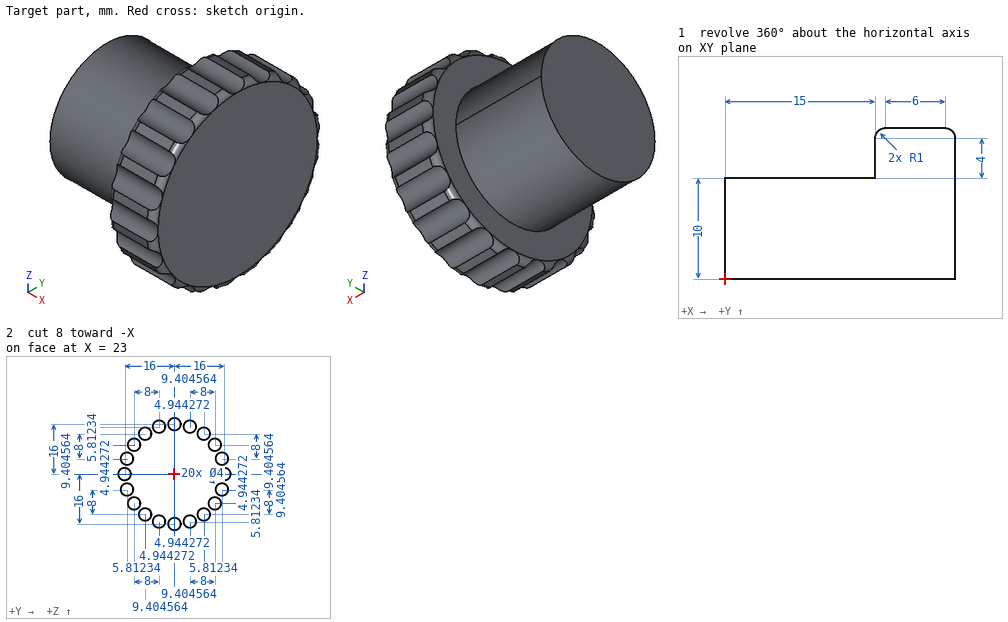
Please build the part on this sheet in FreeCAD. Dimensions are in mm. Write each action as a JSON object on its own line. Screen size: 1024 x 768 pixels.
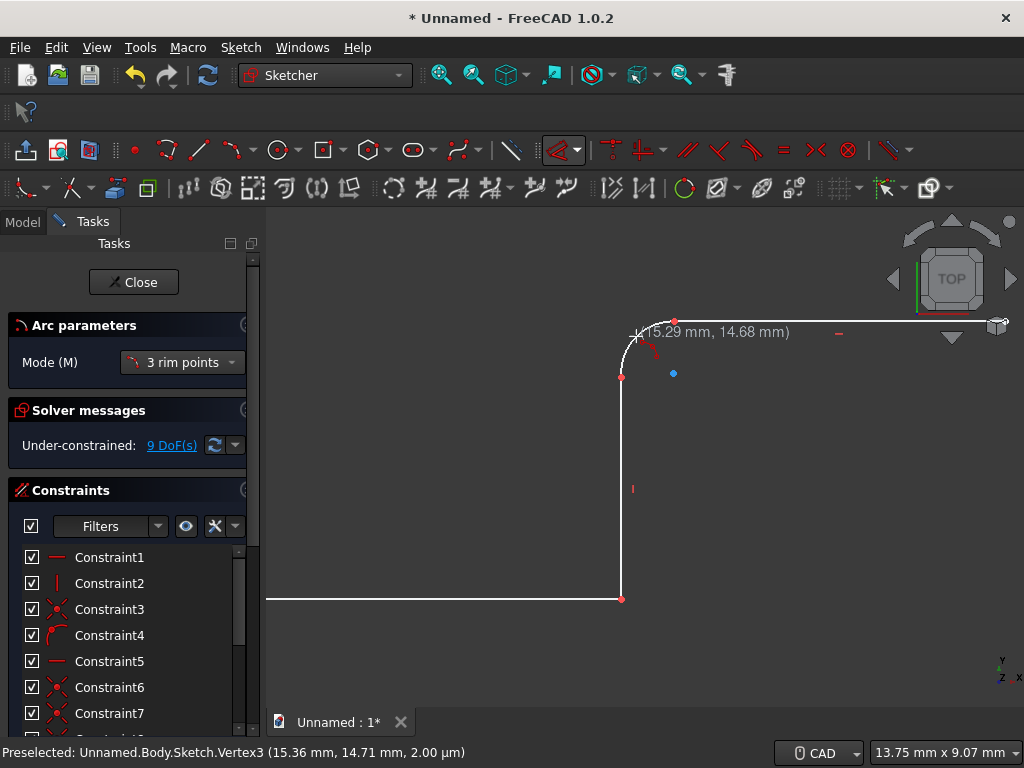
{"action": "scroll", "coordinate": [641, 338], "scroll_direction": "down", "scroll_amount": 6}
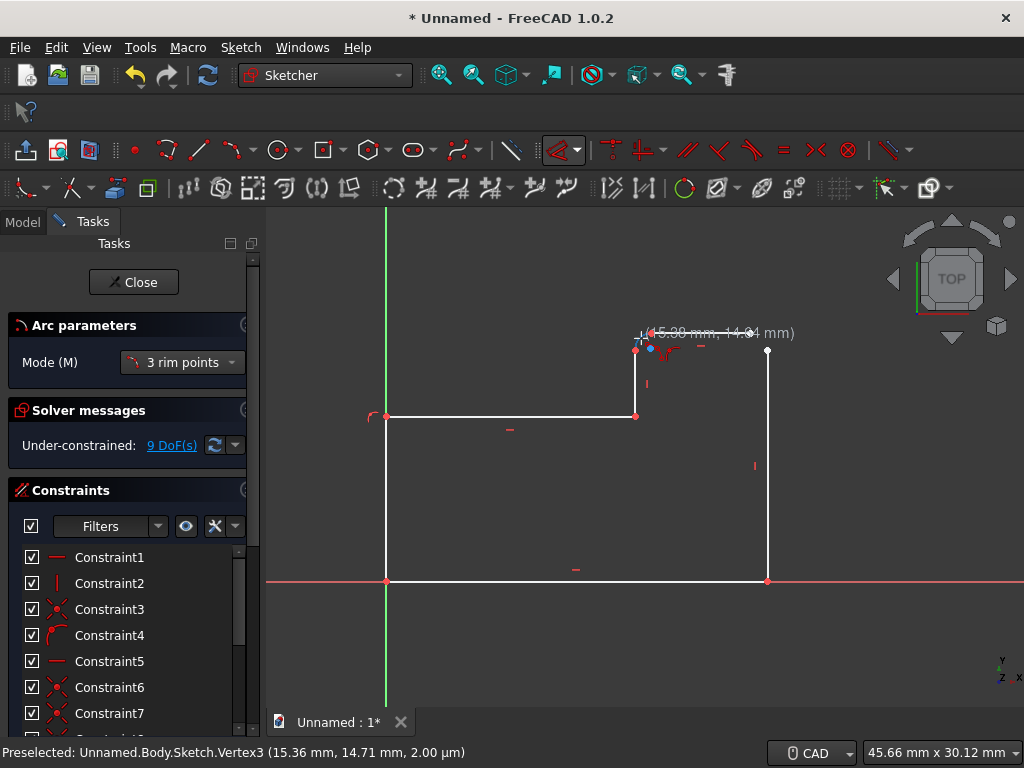
{"action": "left_click", "coordinate": [768, 350]}
{"action": "left_click", "coordinate": [751, 333]}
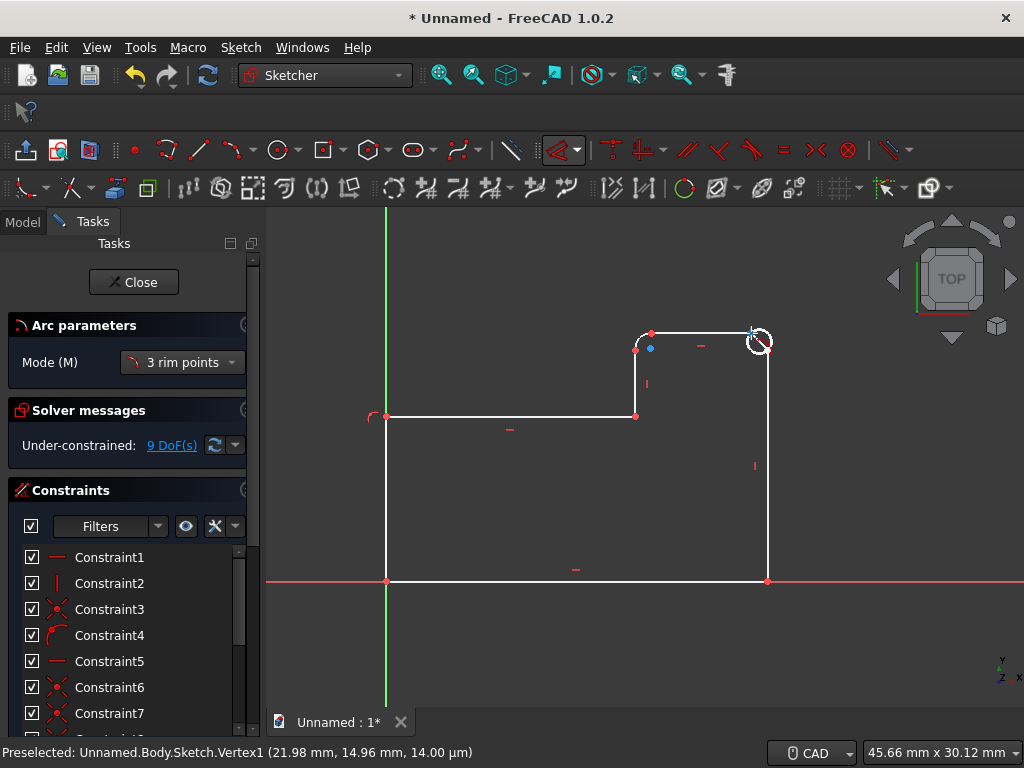
{"action": "scroll", "coordinate": [763, 337], "scroll_direction": "up", "scroll_amount": 6}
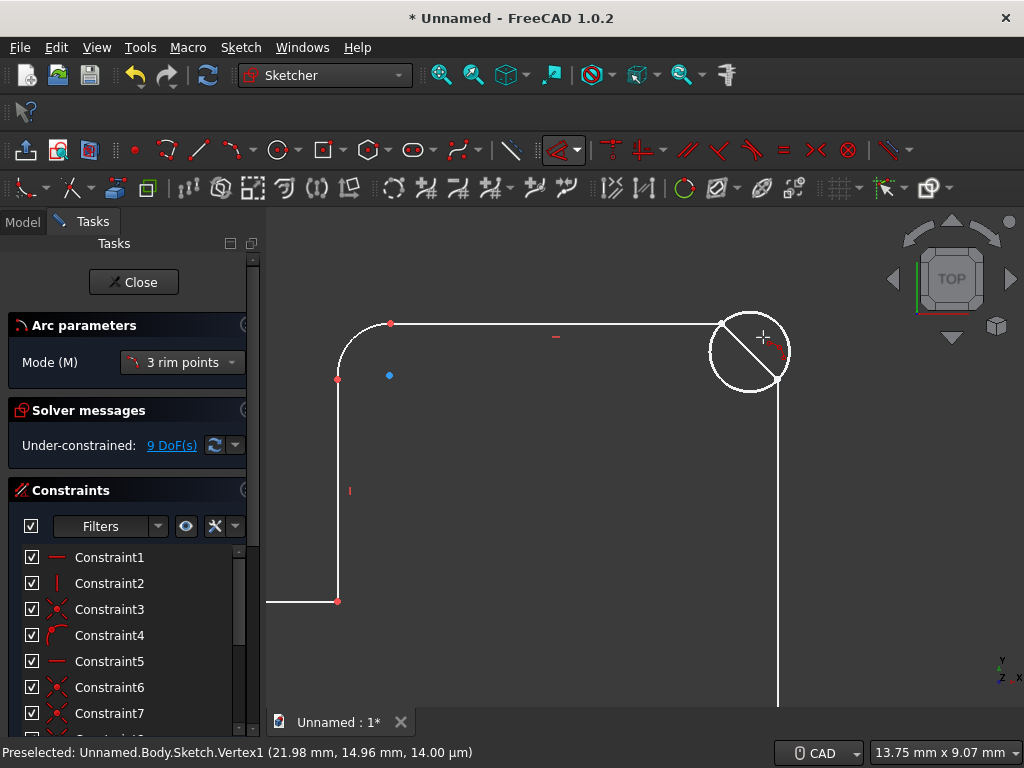
{"action": "left_click", "coordinate": [762, 338]}
{"action": "key", "text": "Escape"}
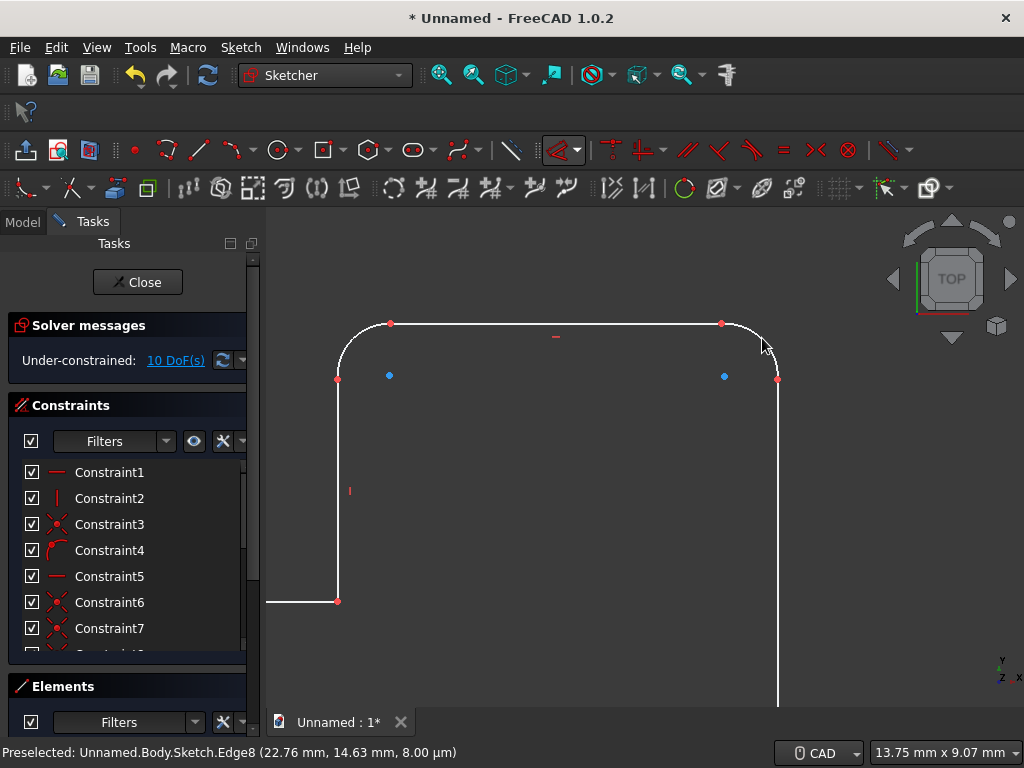
{"action": "left_click", "coordinate": [622, 324]}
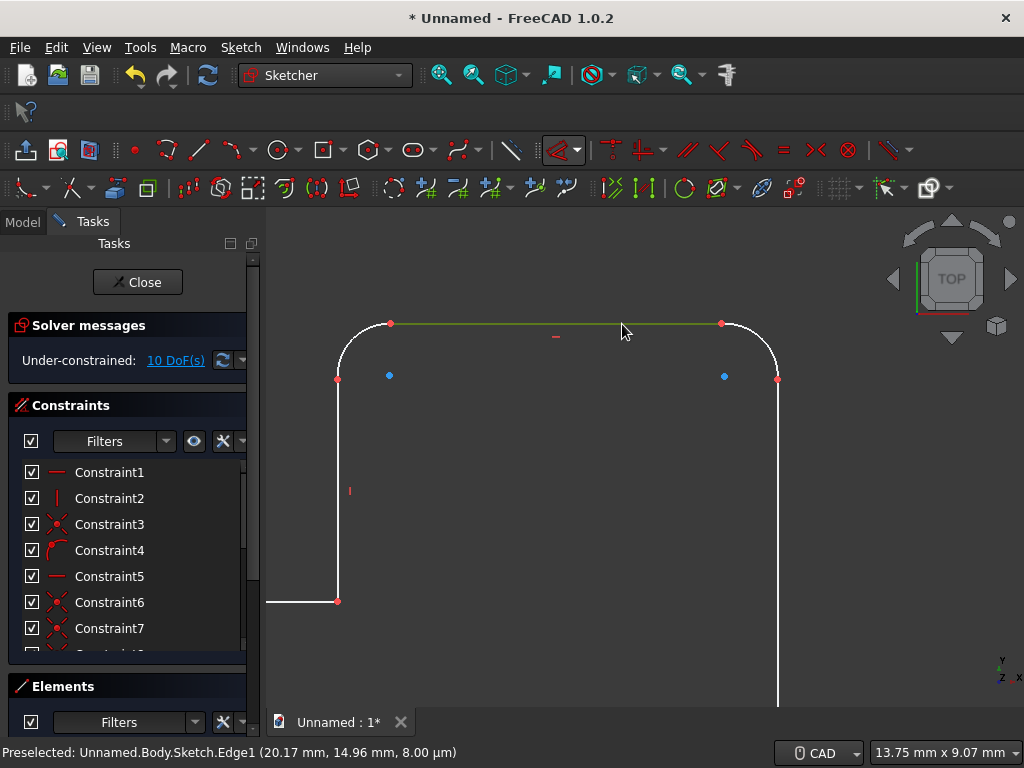
{"action": "left_click", "coordinate": [366, 330]}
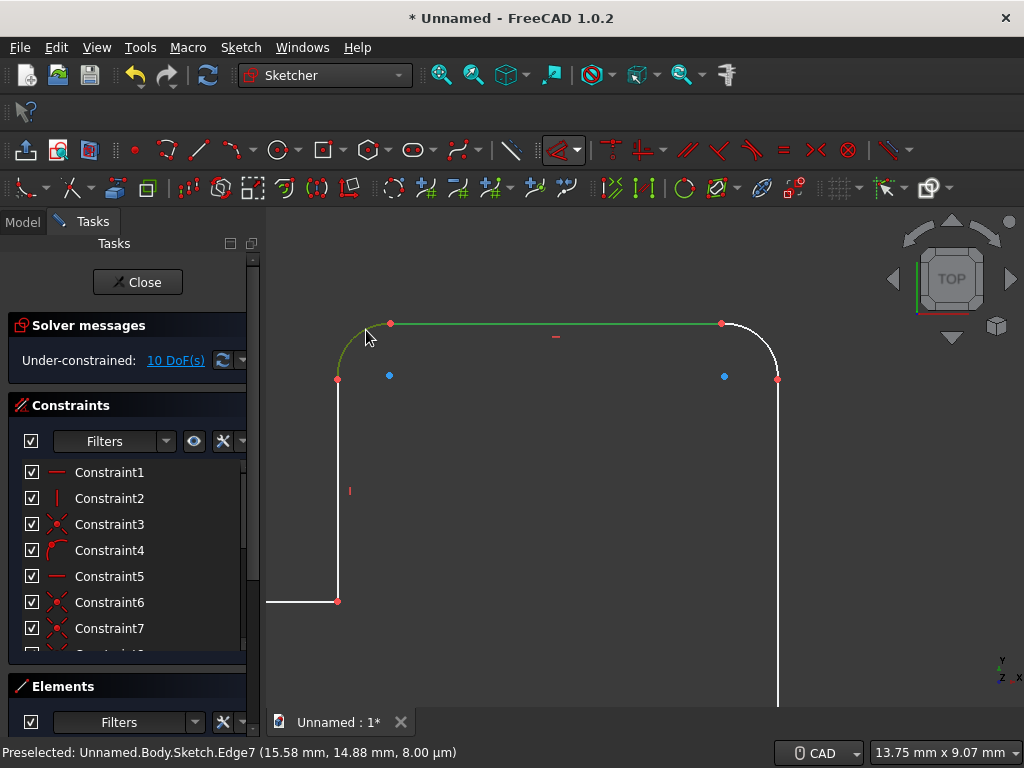
{"action": "left_click", "coordinate": [752, 150]}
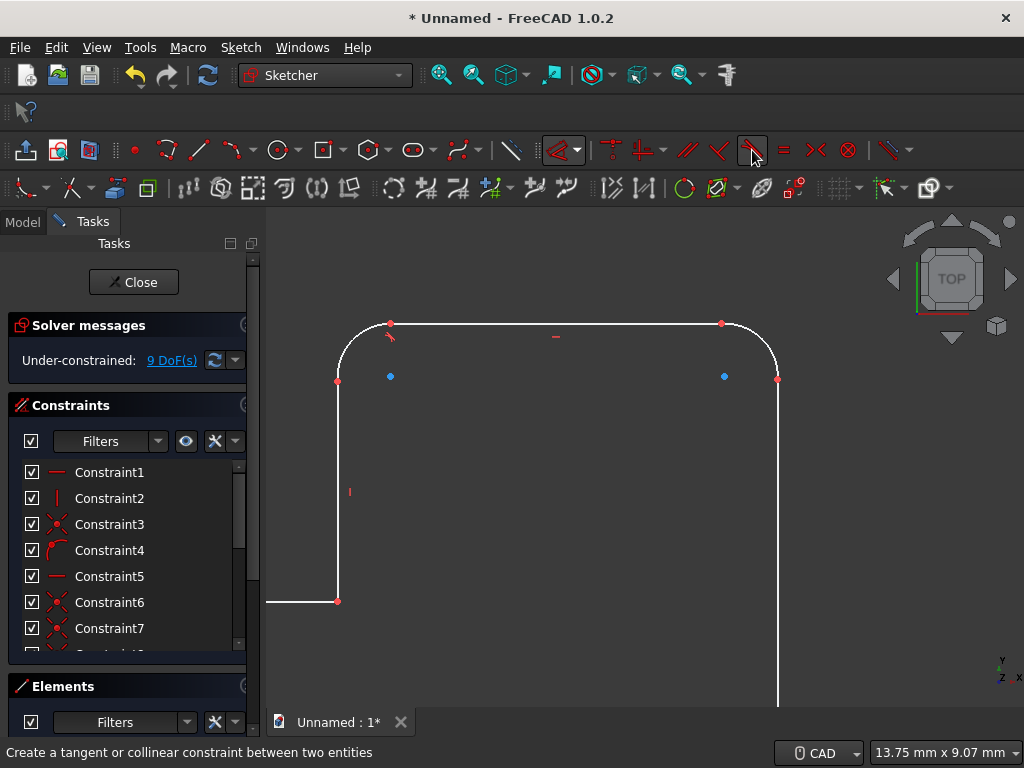
{"action": "left_click", "coordinate": [622, 324]}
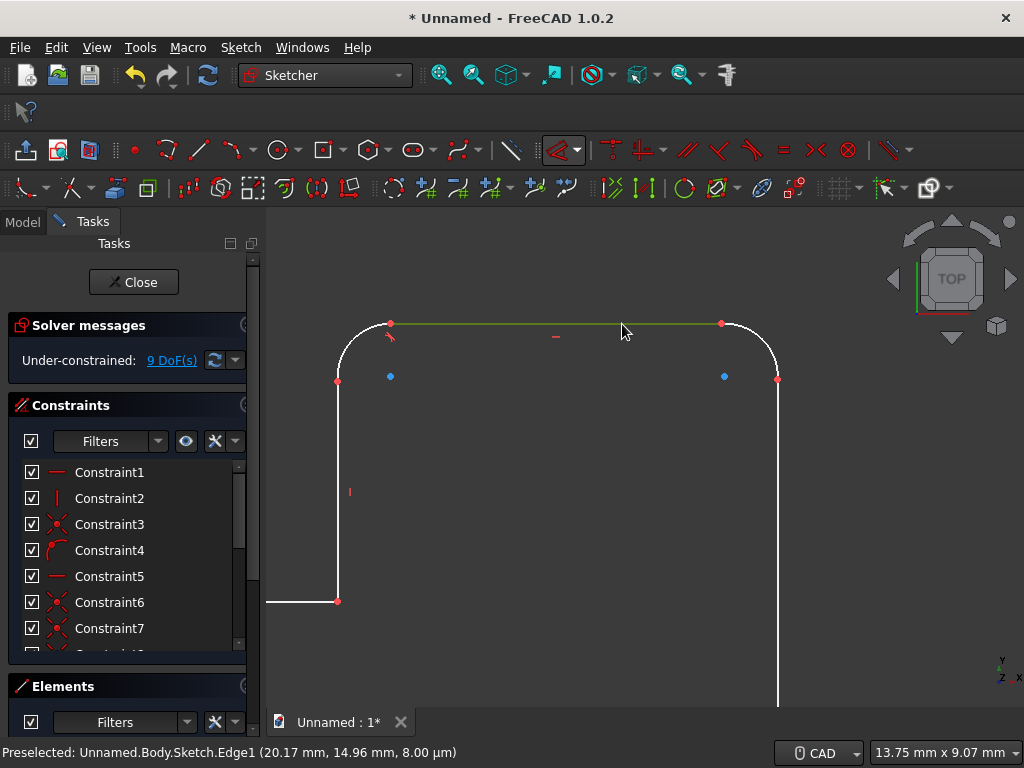
{"action": "left_click", "coordinate": [773, 354]}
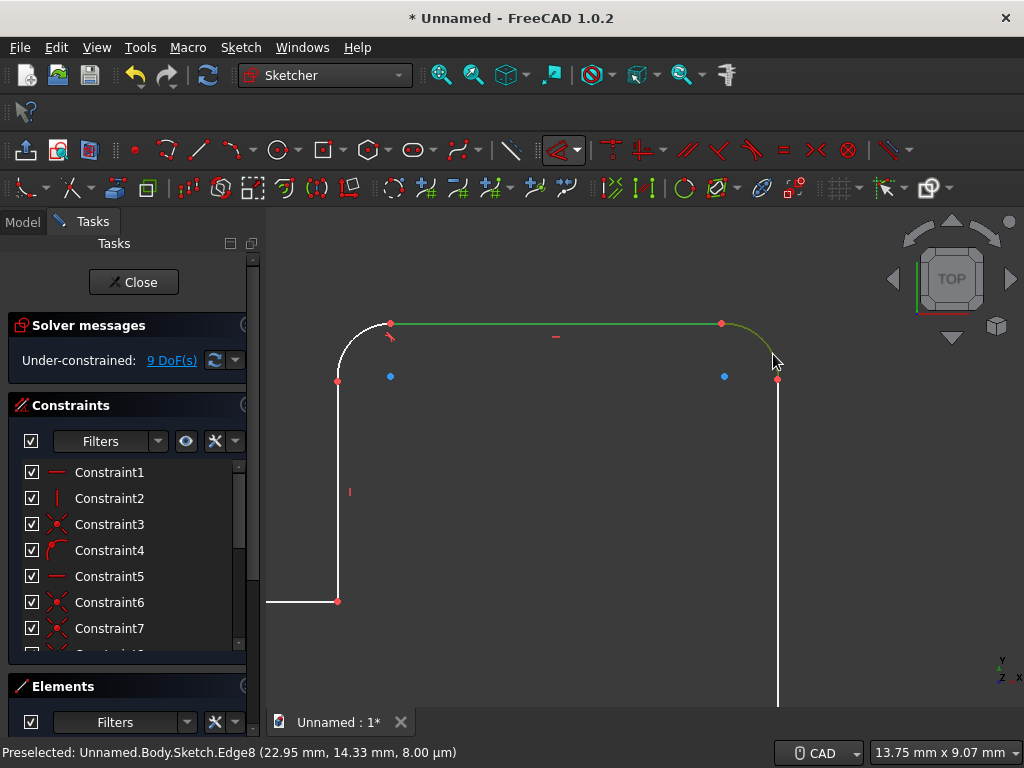
{"action": "left_click", "coordinate": [752, 150]}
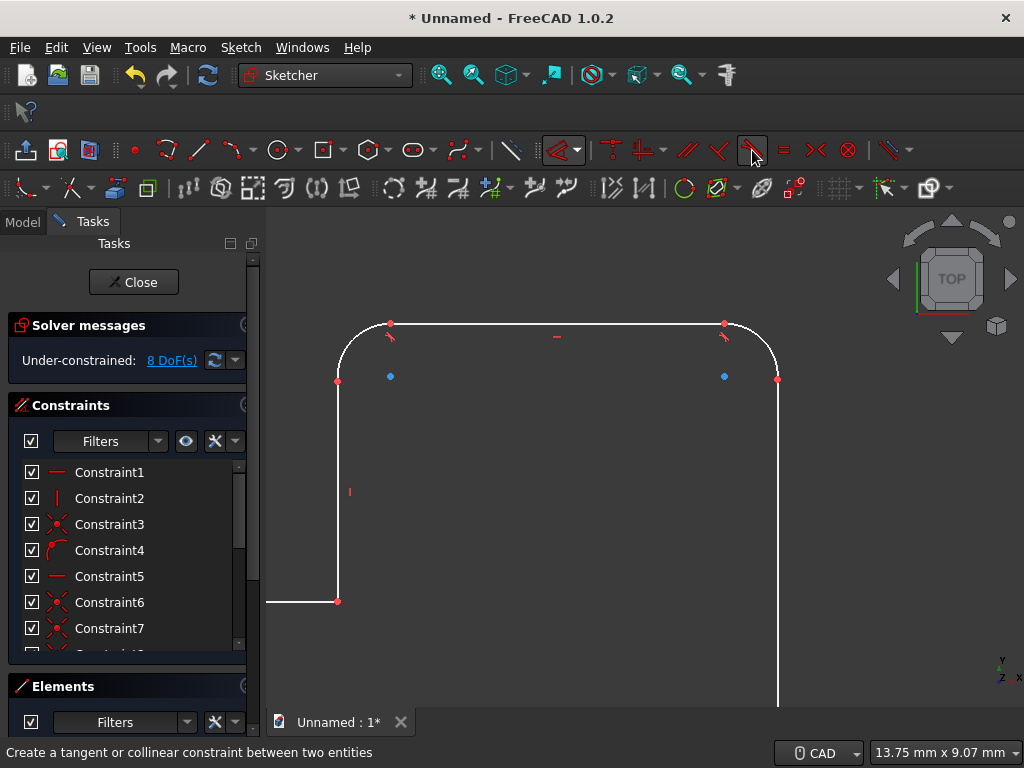
{"action": "left_click", "coordinate": [338, 447]}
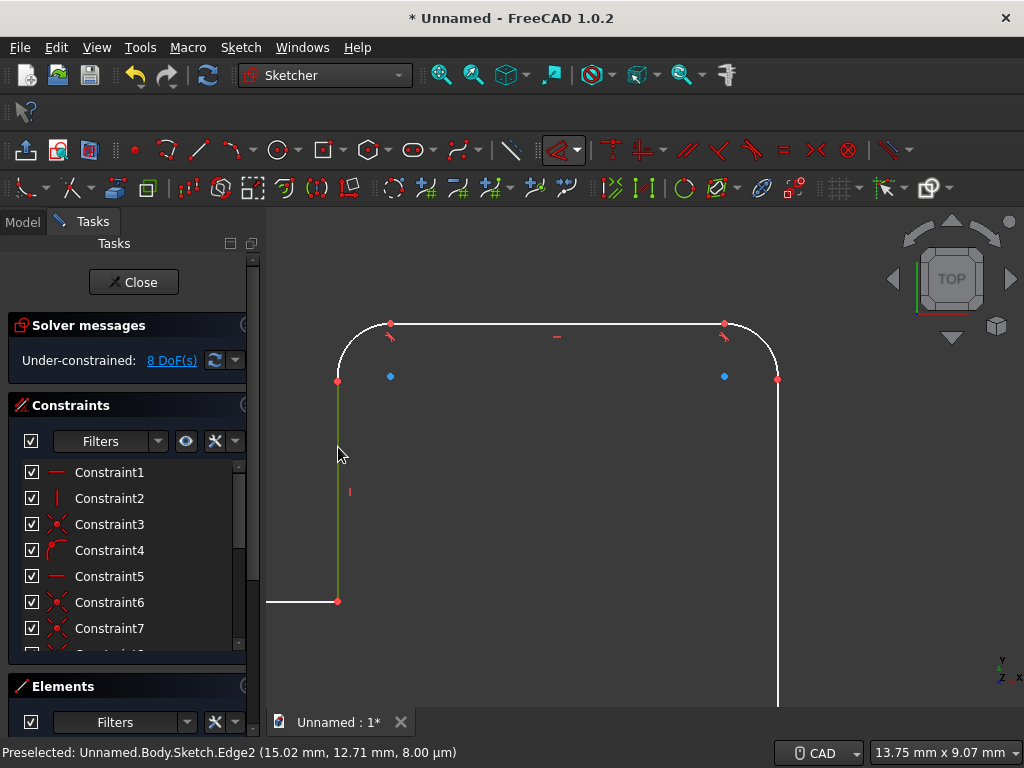
{"action": "left_click", "coordinate": [366, 330]}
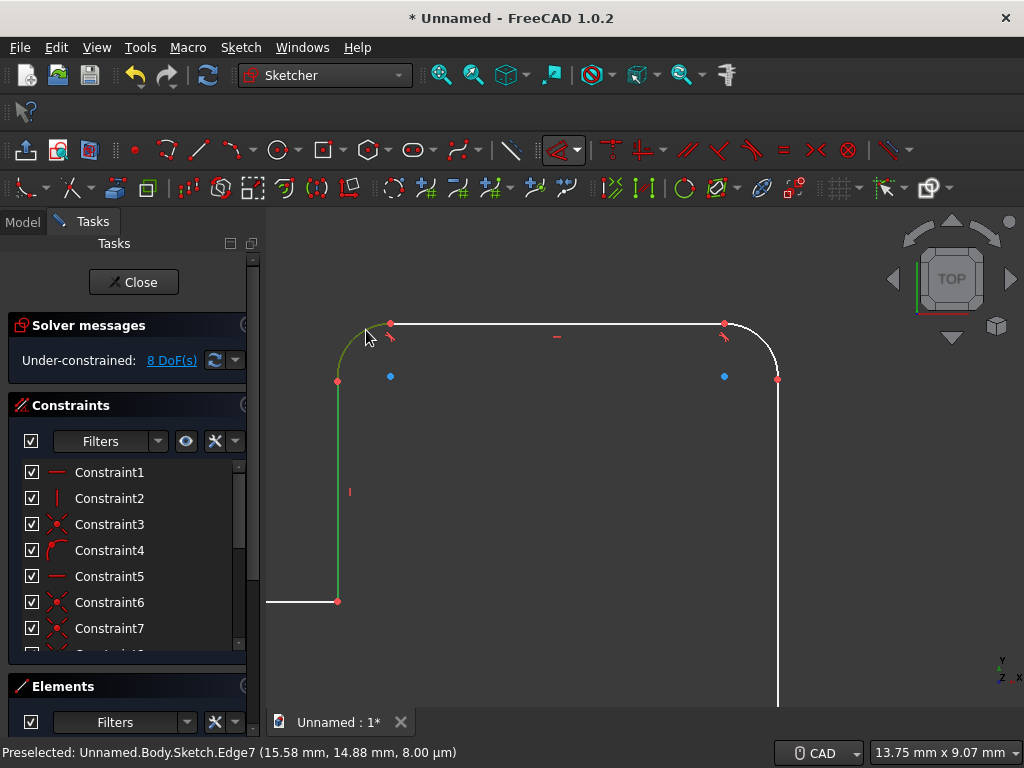
{"action": "left_click", "coordinate": [752, 150]}